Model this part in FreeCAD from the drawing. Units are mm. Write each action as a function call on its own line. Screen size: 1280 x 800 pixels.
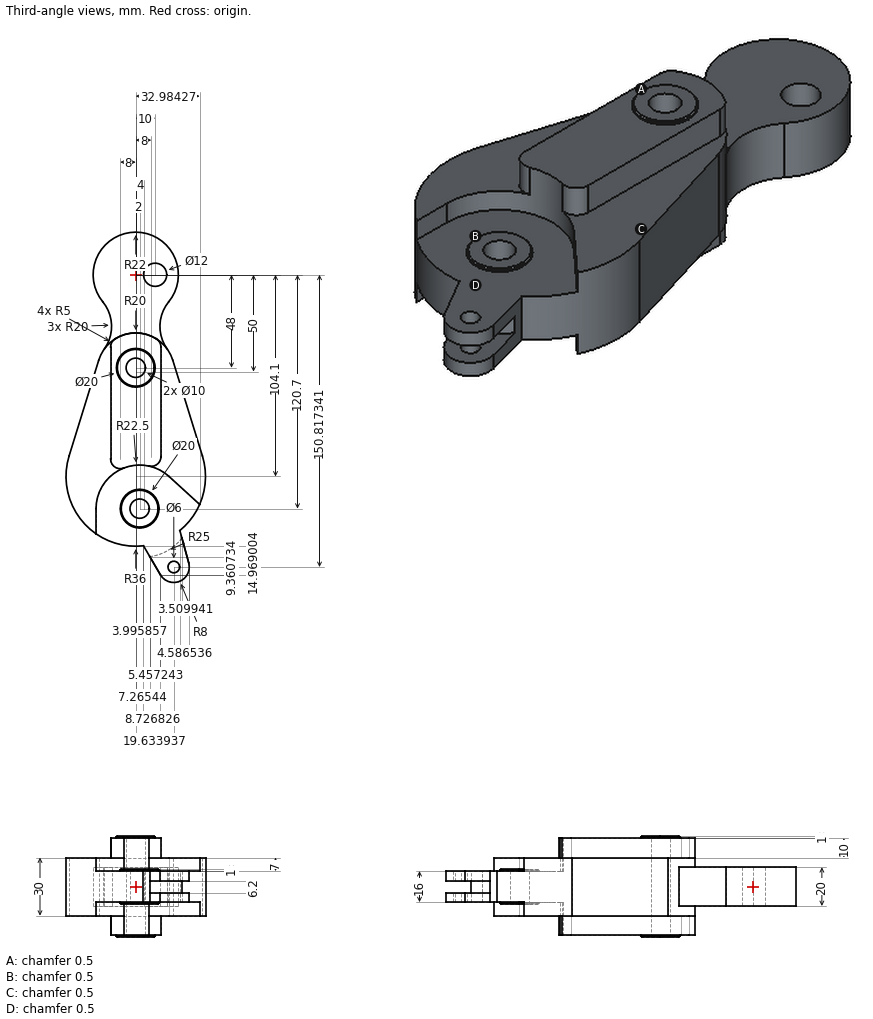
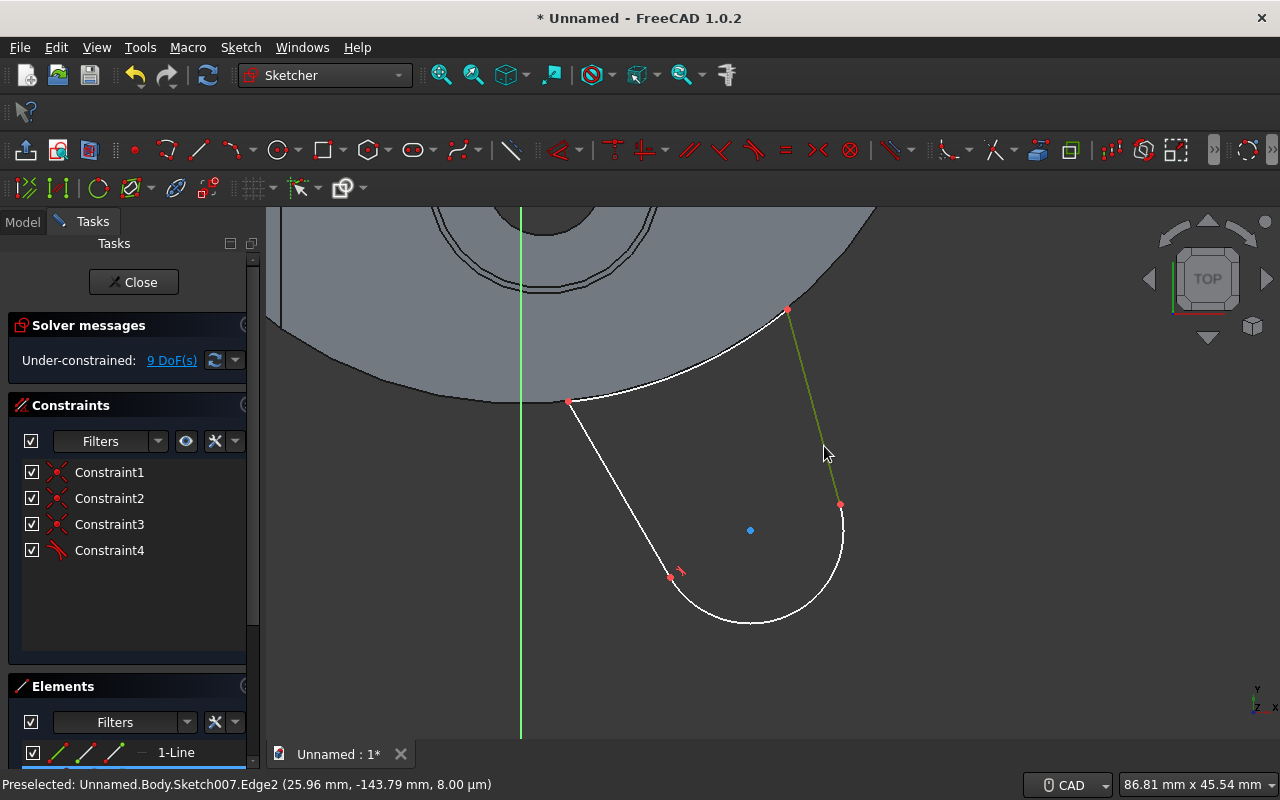
click(734, 622)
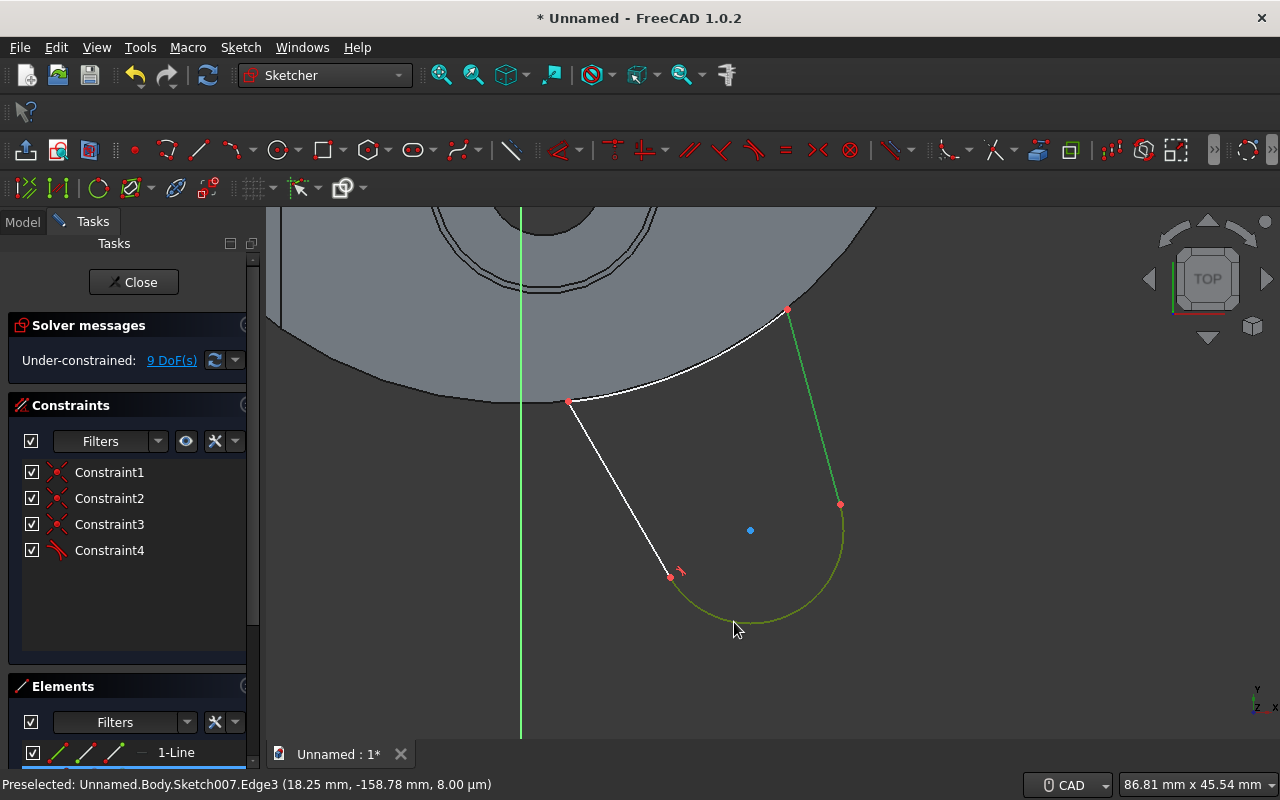
click(754, 150)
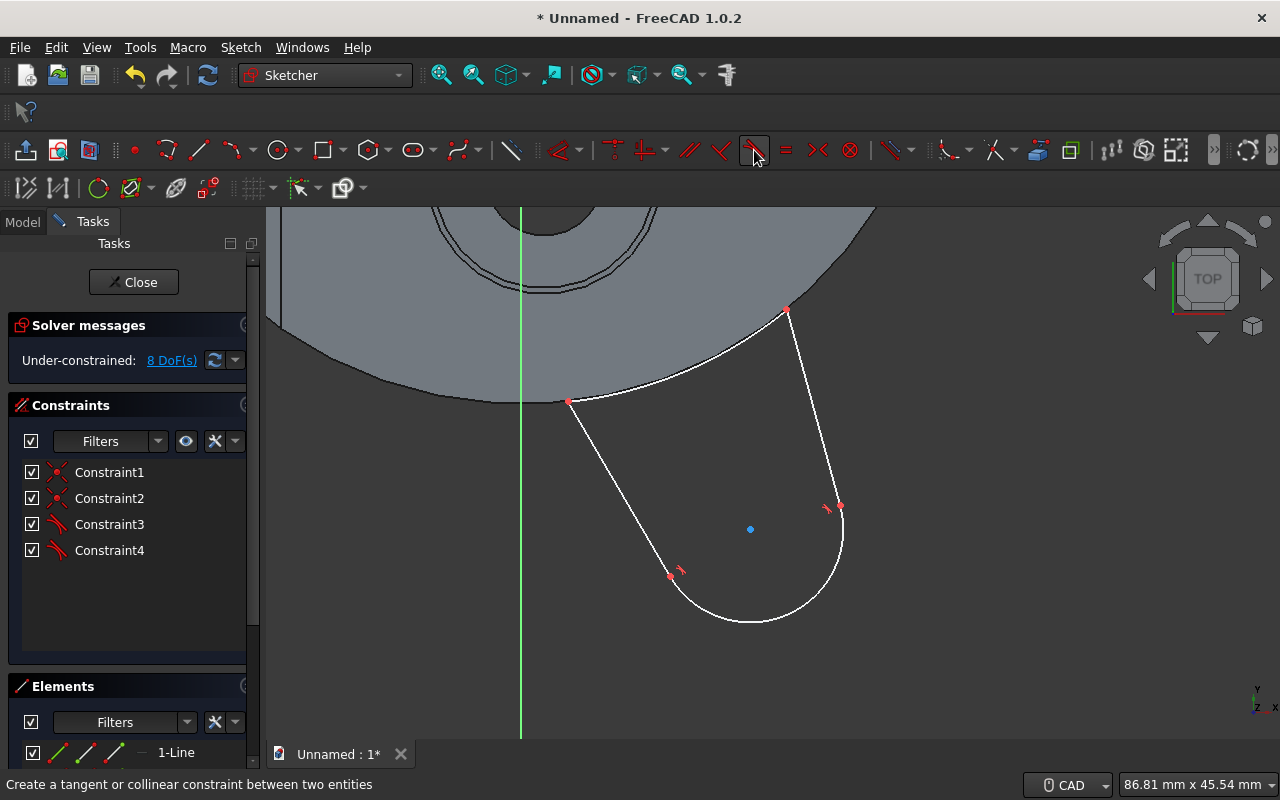
scroll(732, 682, down, 3)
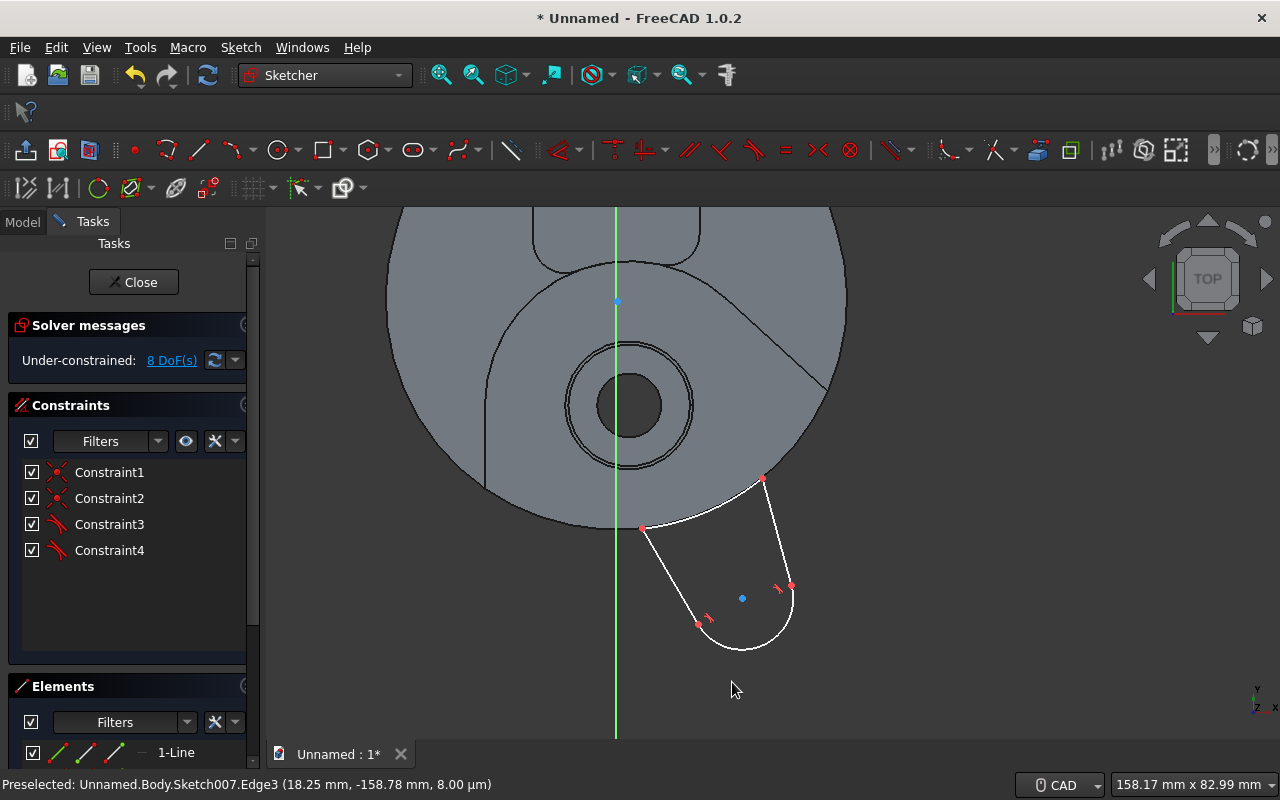
click(617, 301)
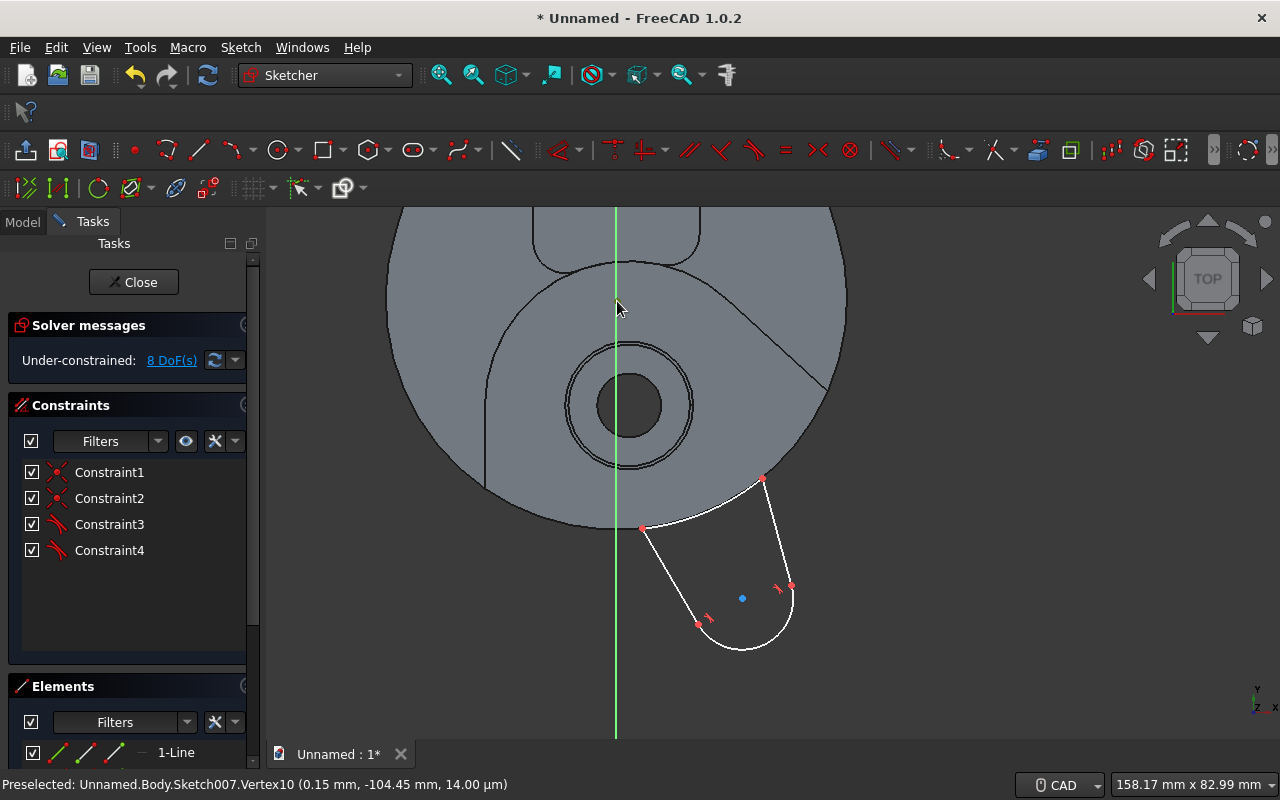
click(616, 677)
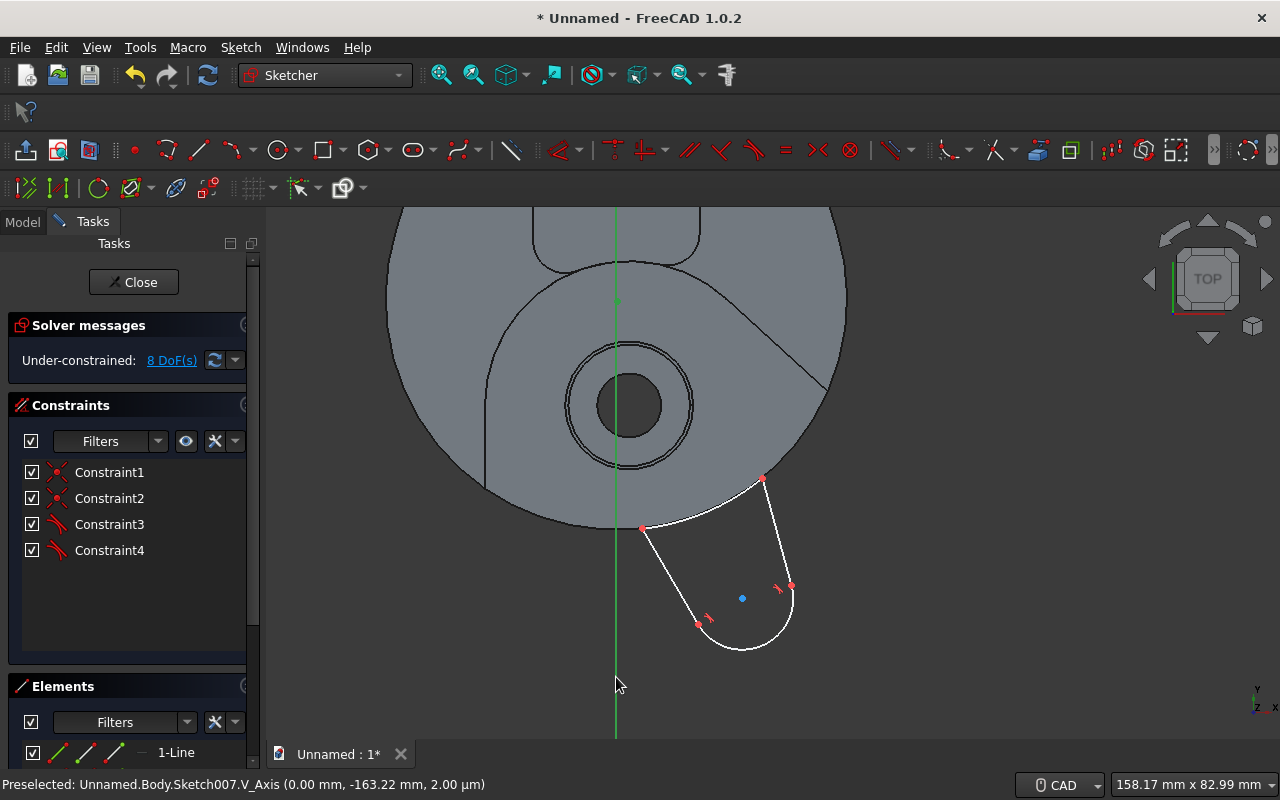
click(614, 150)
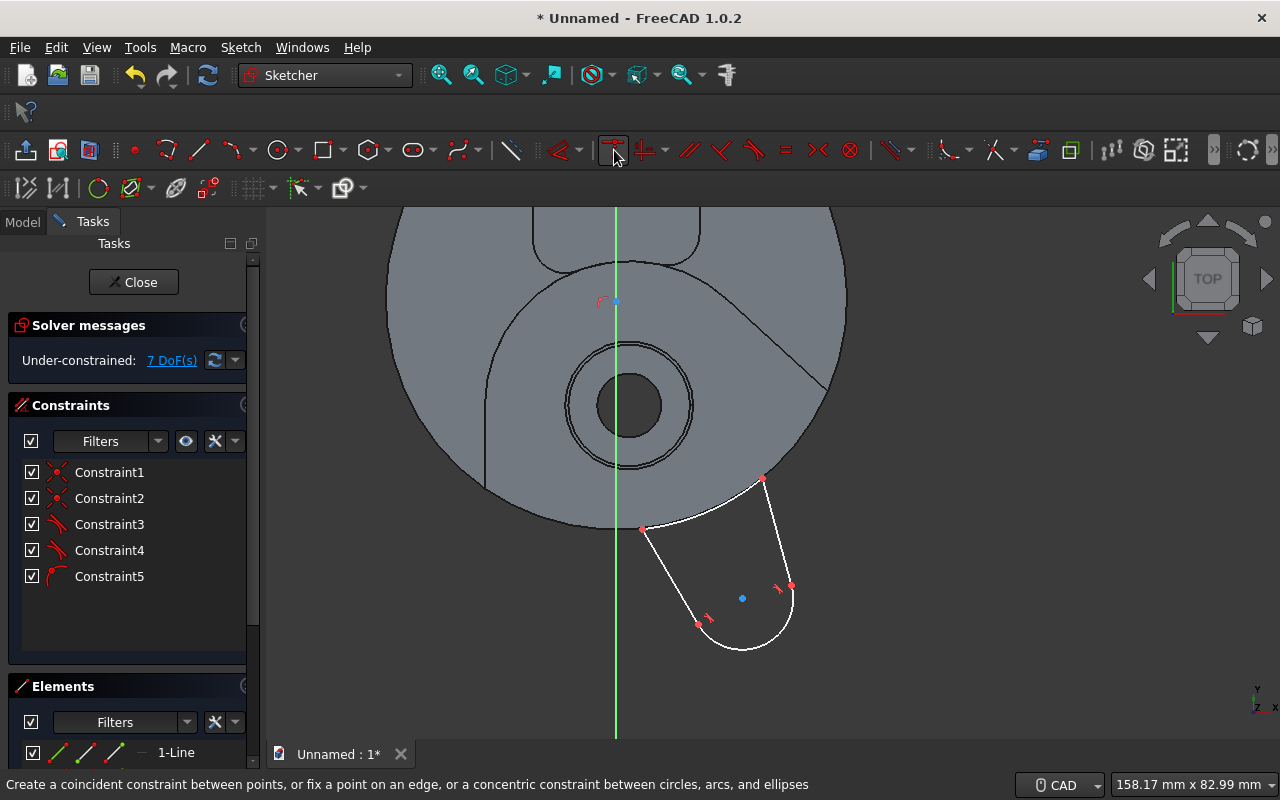
click(558, 150)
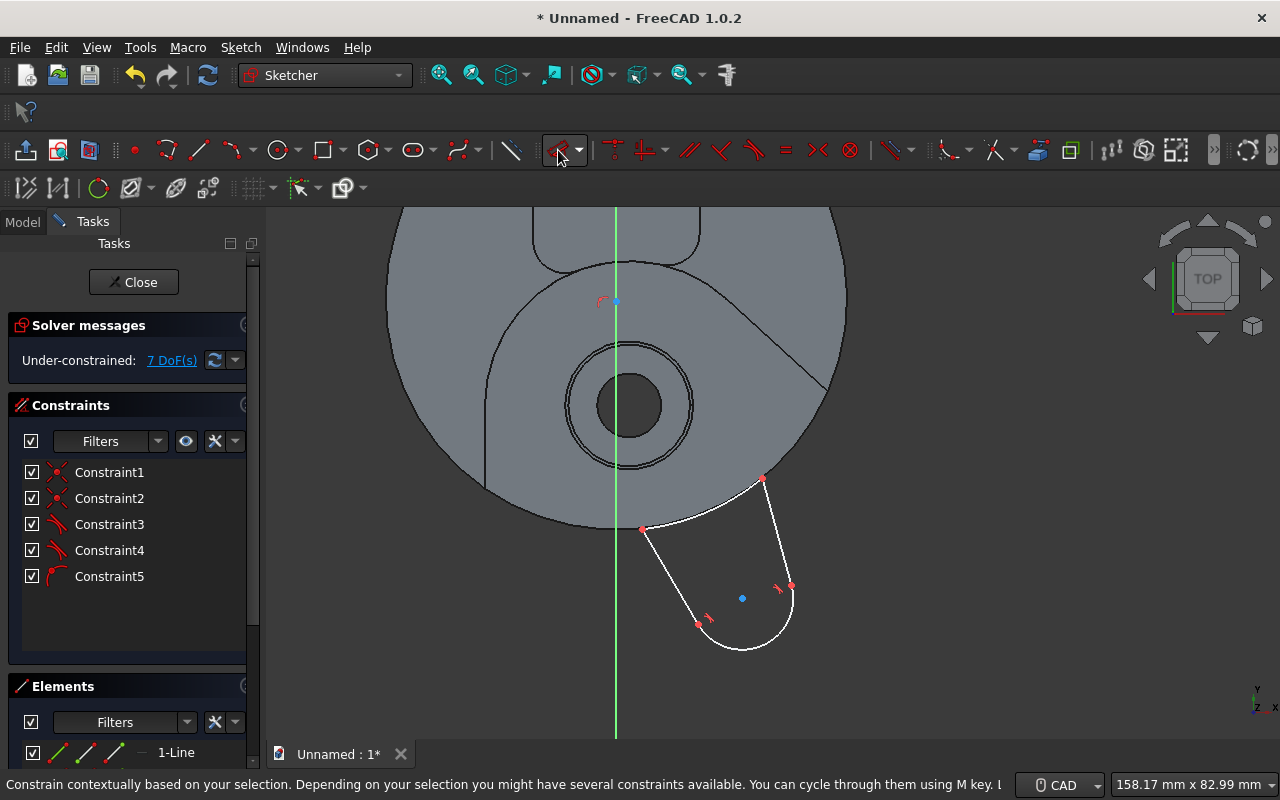
click(733, 649)
click(727, 680)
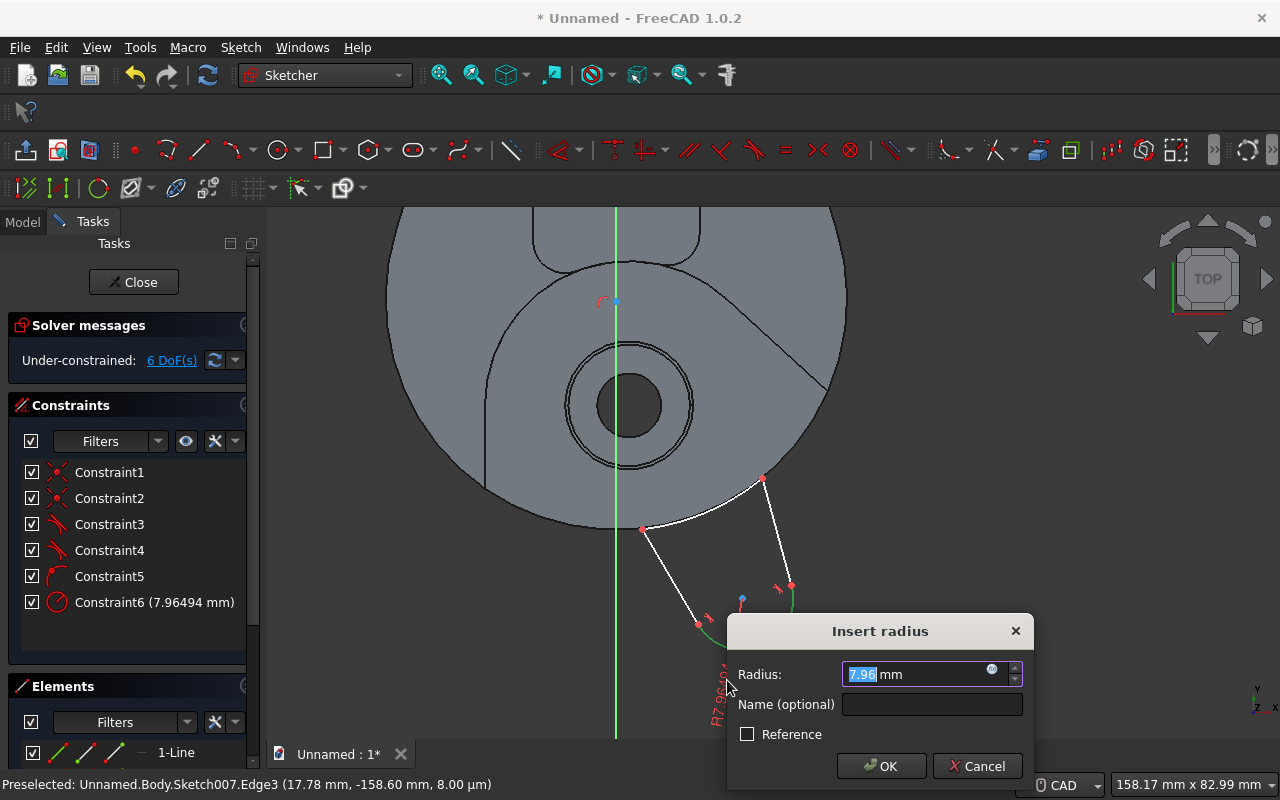
text(8)
key(Return)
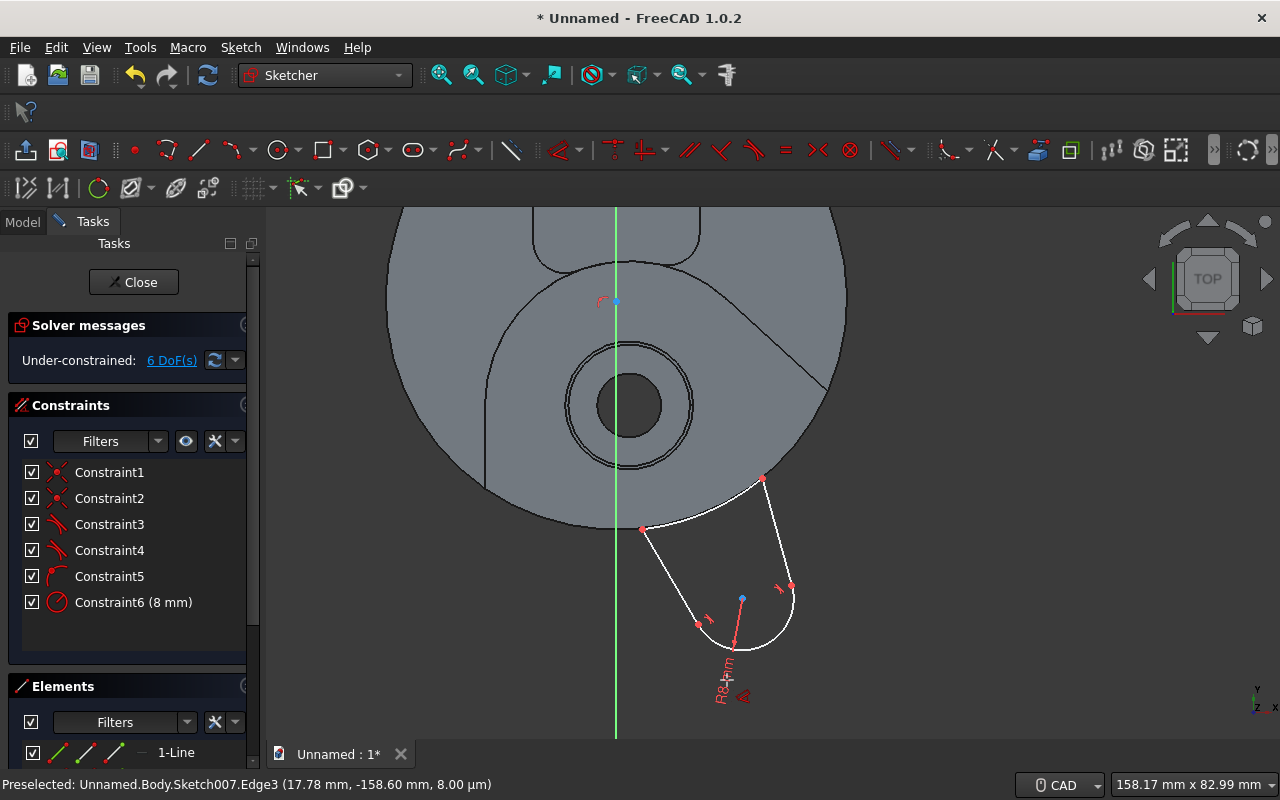
click(681, 521)
click(690, 552)